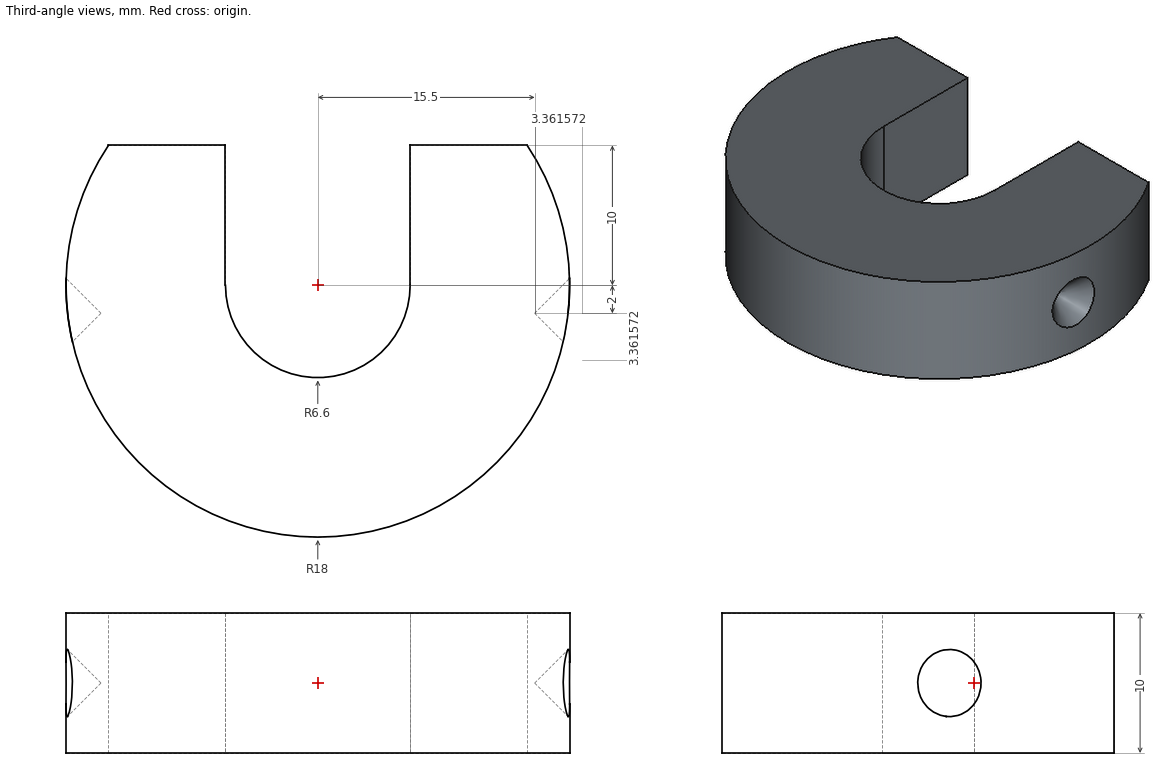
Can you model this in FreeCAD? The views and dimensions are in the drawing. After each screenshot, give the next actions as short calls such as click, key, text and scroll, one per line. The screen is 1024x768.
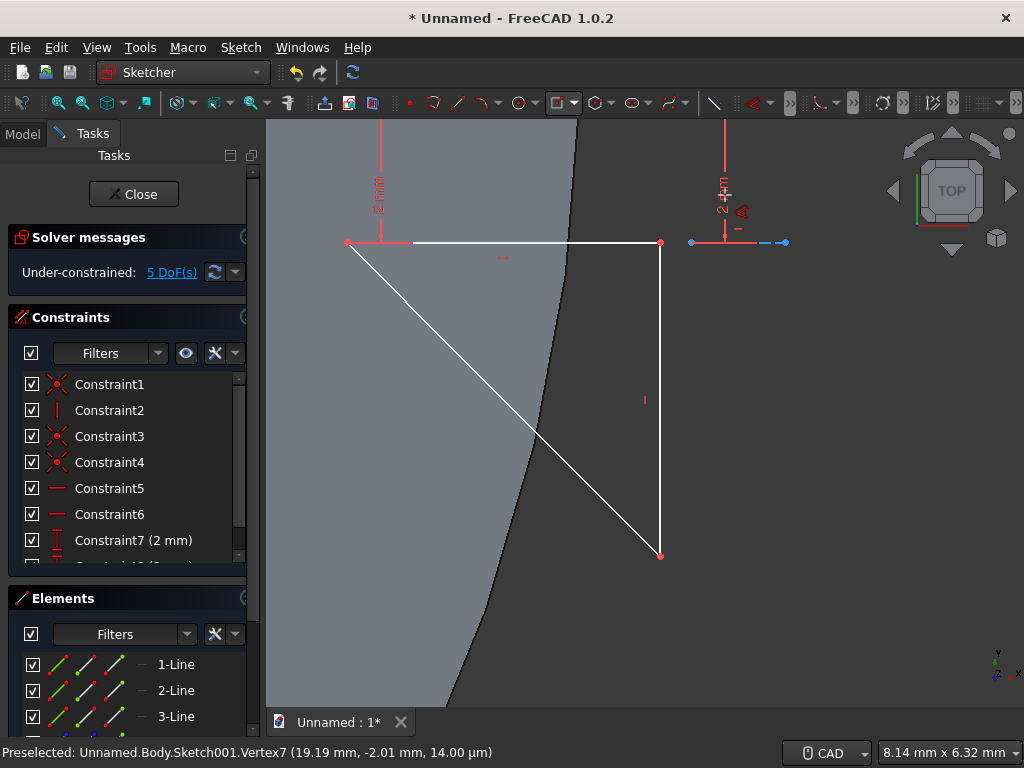
click(347, 243)
click(320, 277)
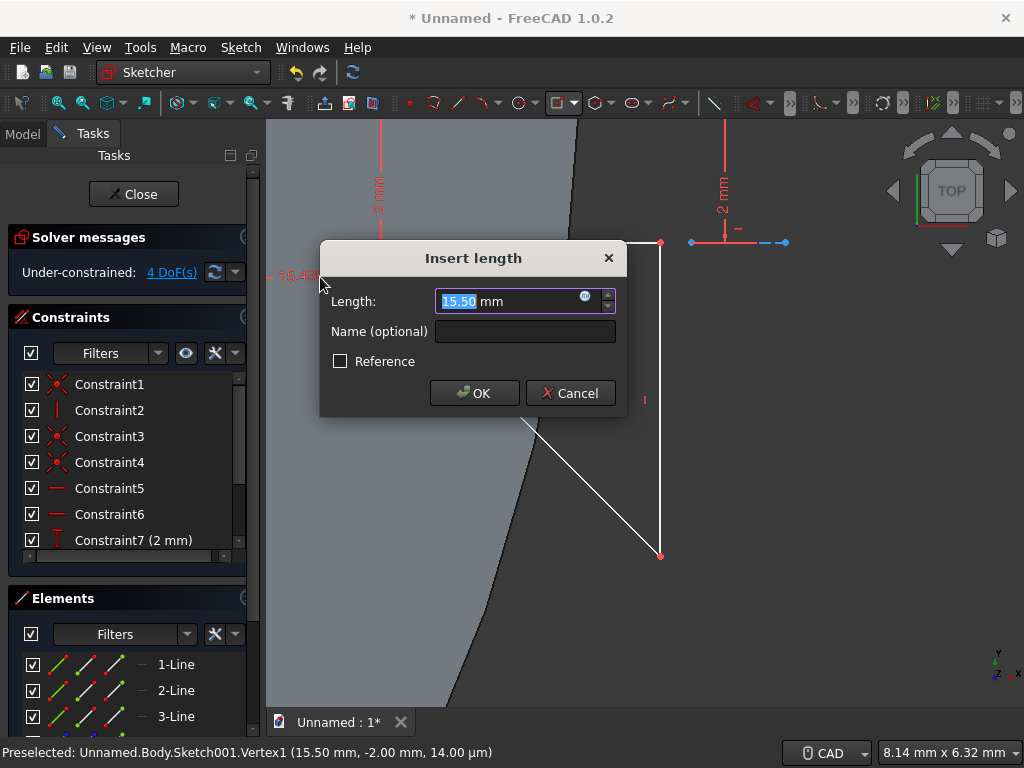
text(15.5)
key(Return)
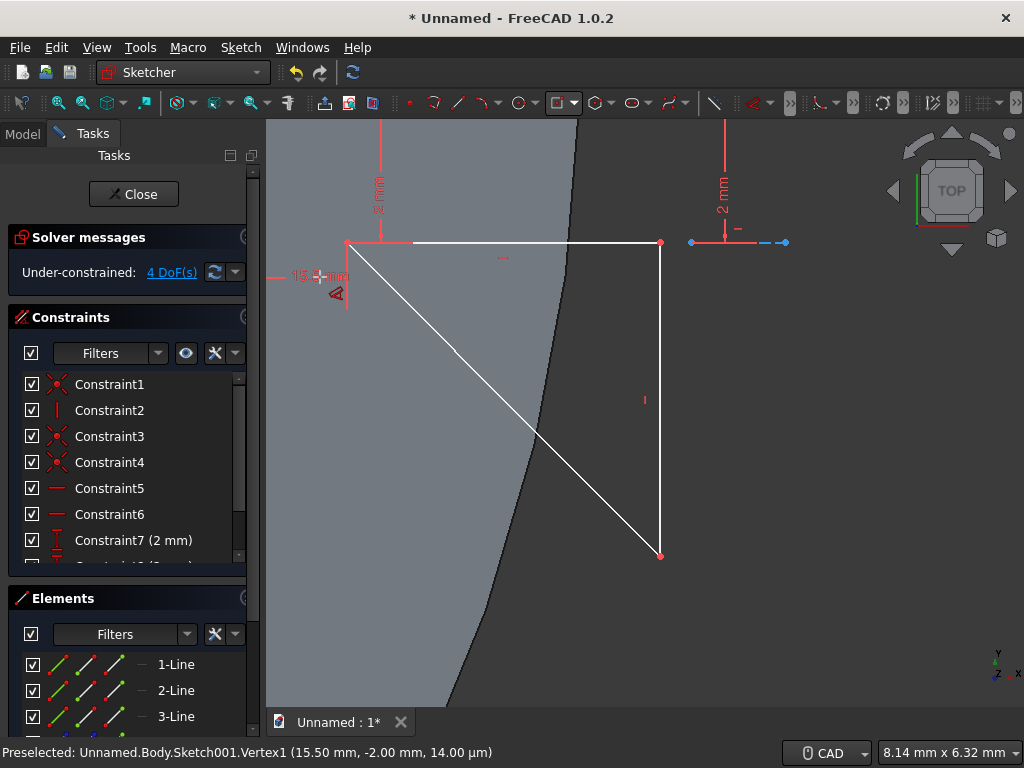
click(660, 463)
click(694, 400)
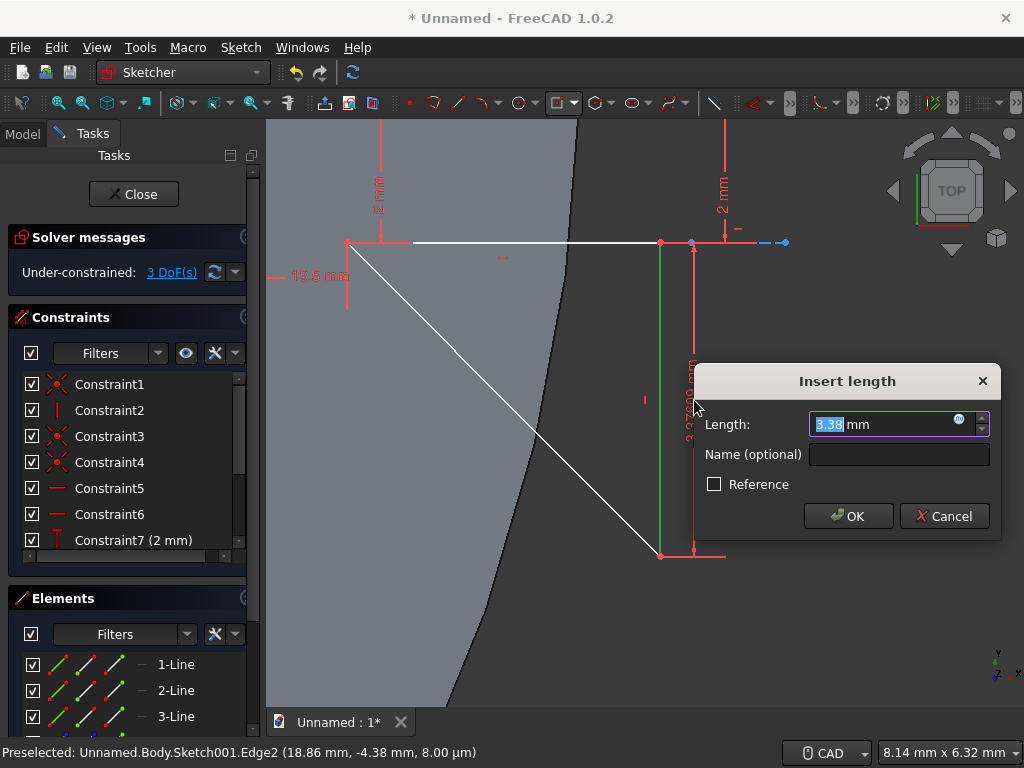
text(3.361572)
key(Return)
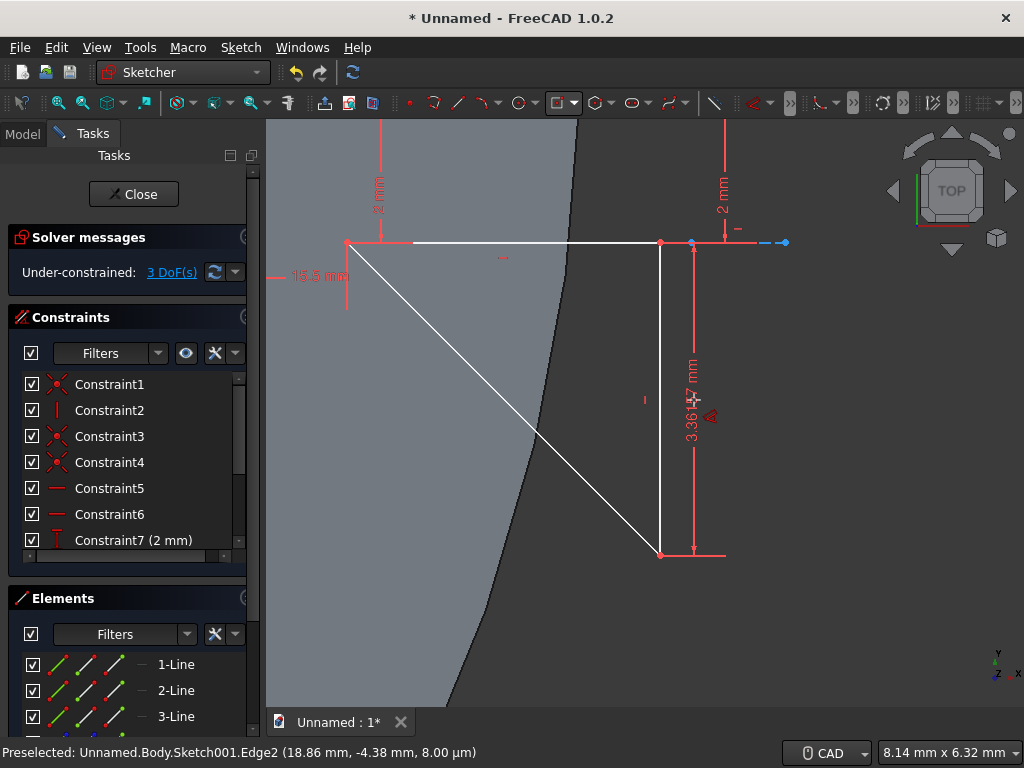
click(566, 243)
click(504, 209)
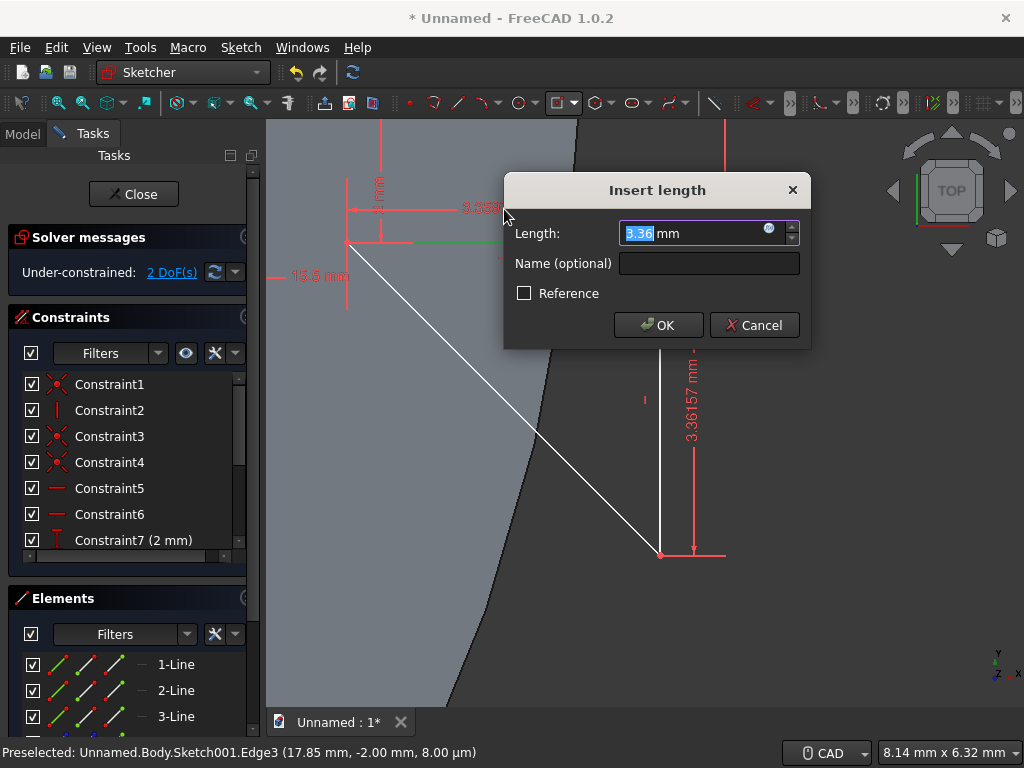
text(3.361572)
key(Return)
key(Escape)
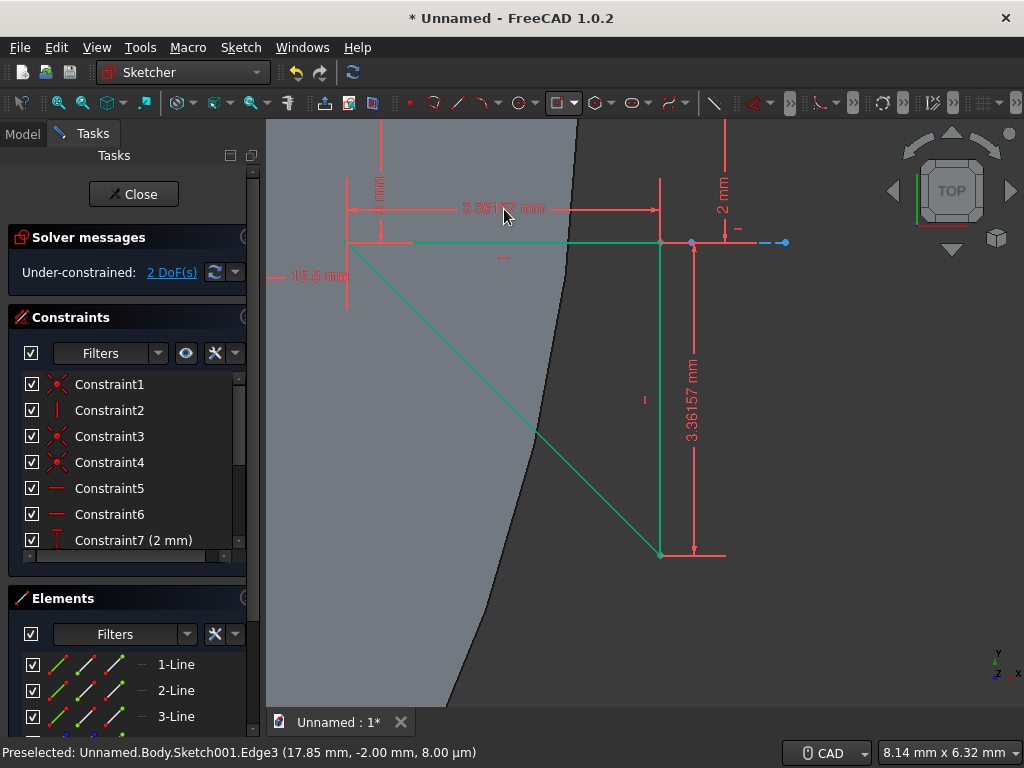
click(134, 194)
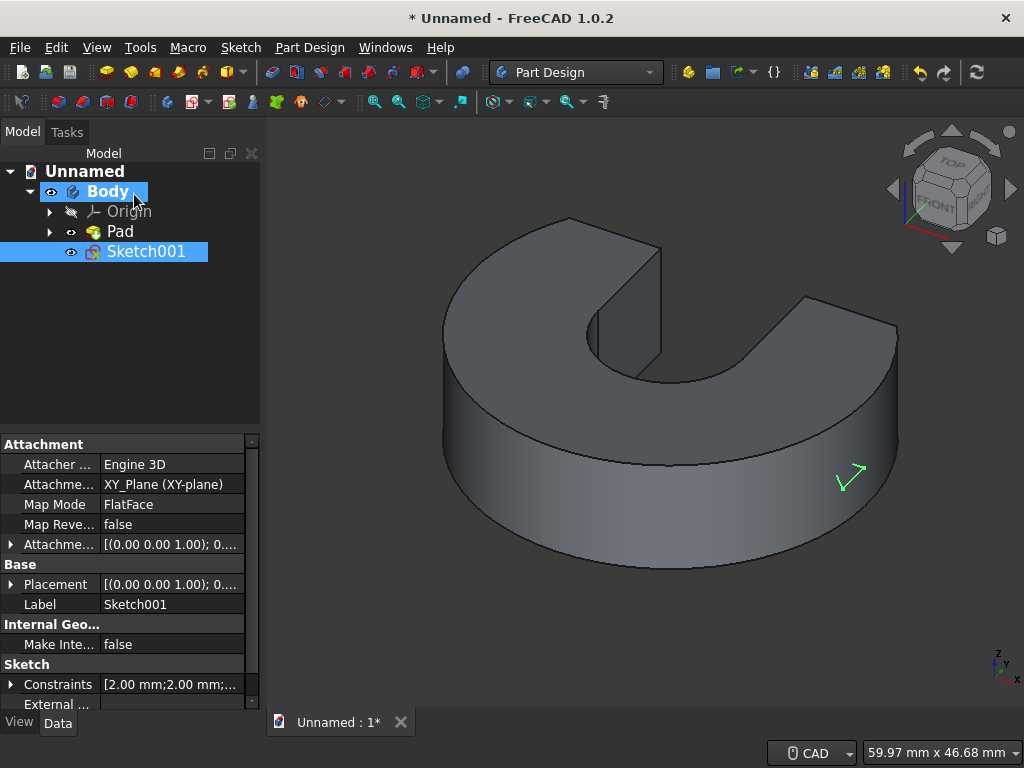
click(322, 72)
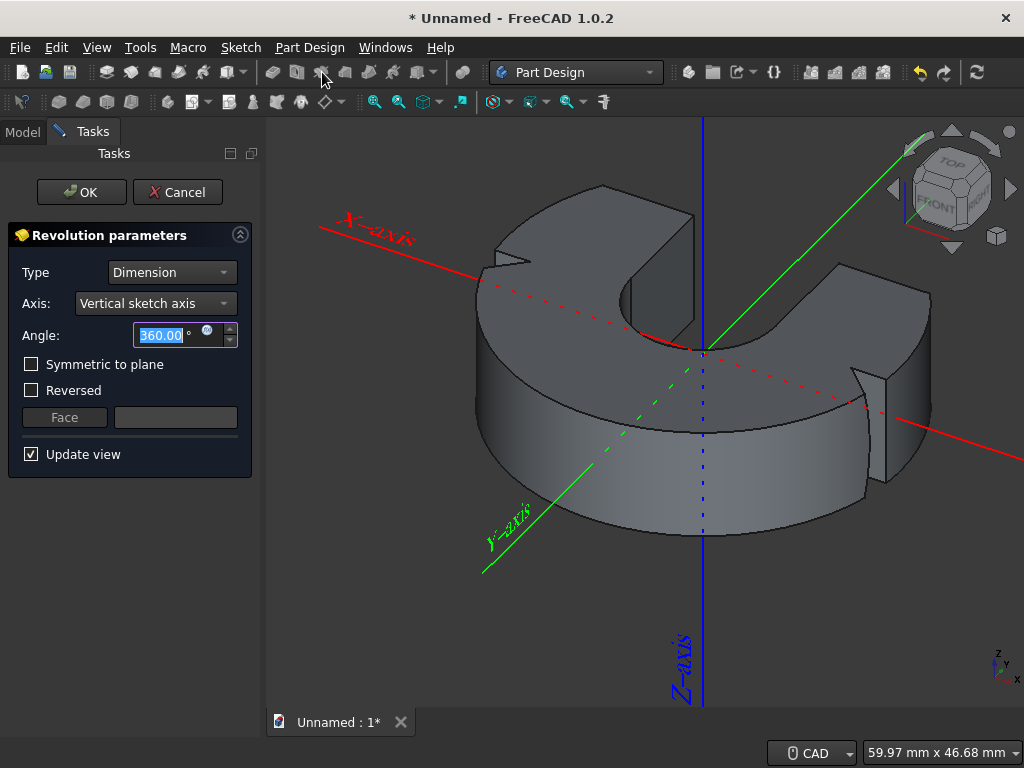
click(156, 304)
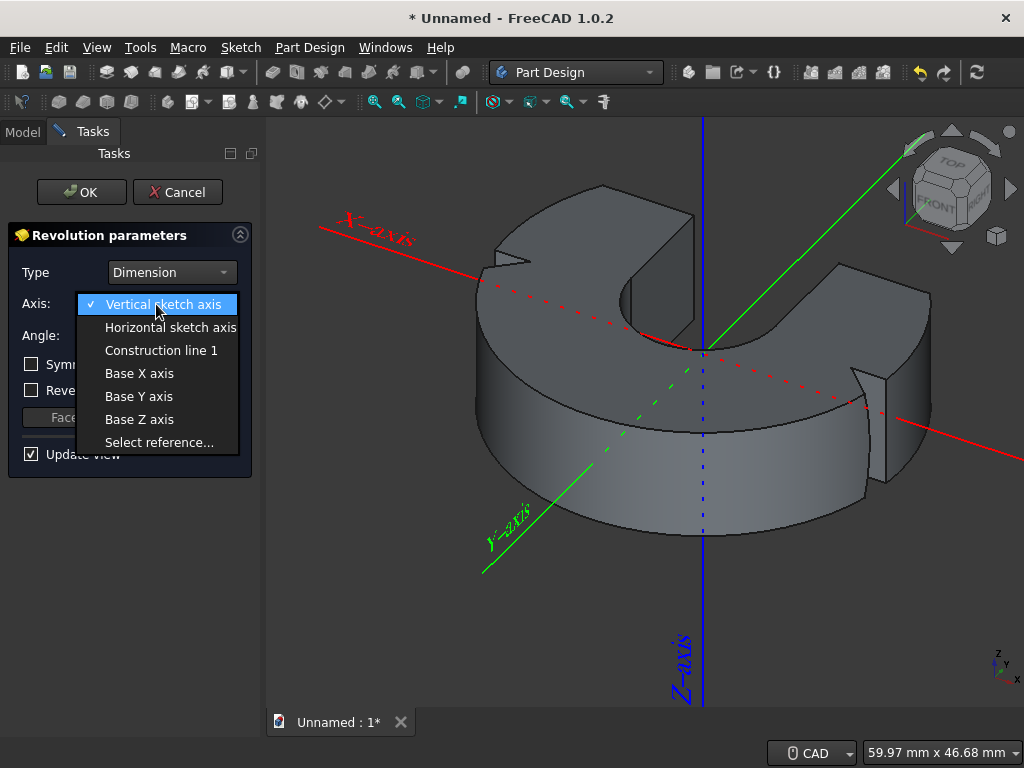
click(156, 350)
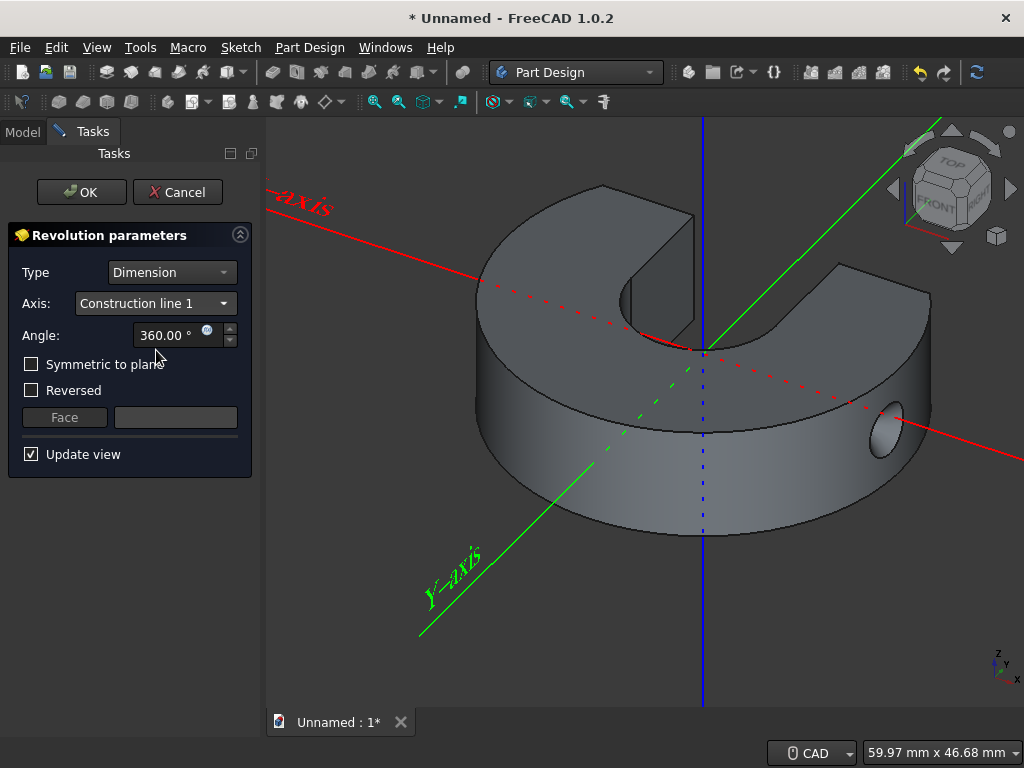
click(82, 192)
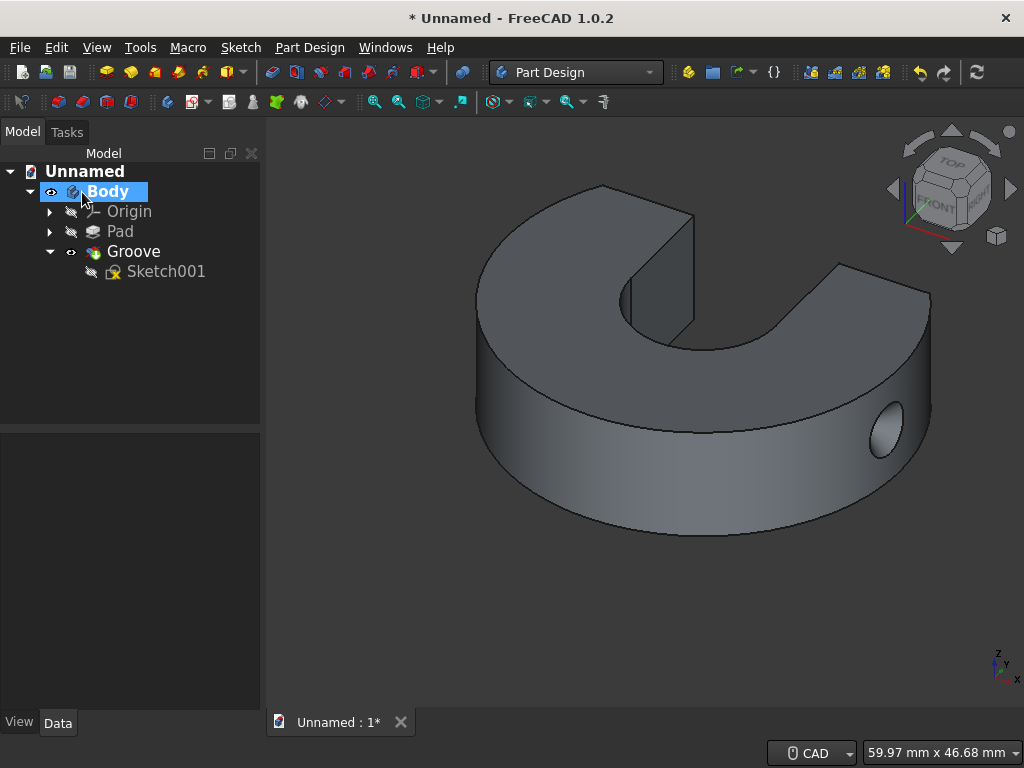
click(116, 252)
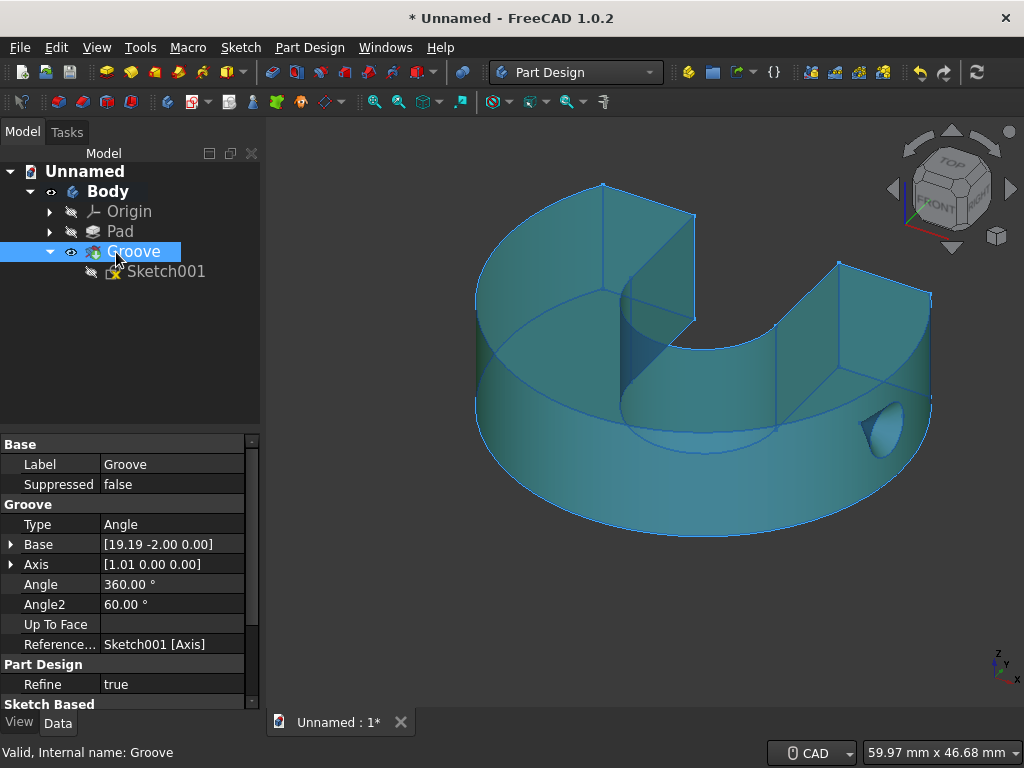
click(812, 72)